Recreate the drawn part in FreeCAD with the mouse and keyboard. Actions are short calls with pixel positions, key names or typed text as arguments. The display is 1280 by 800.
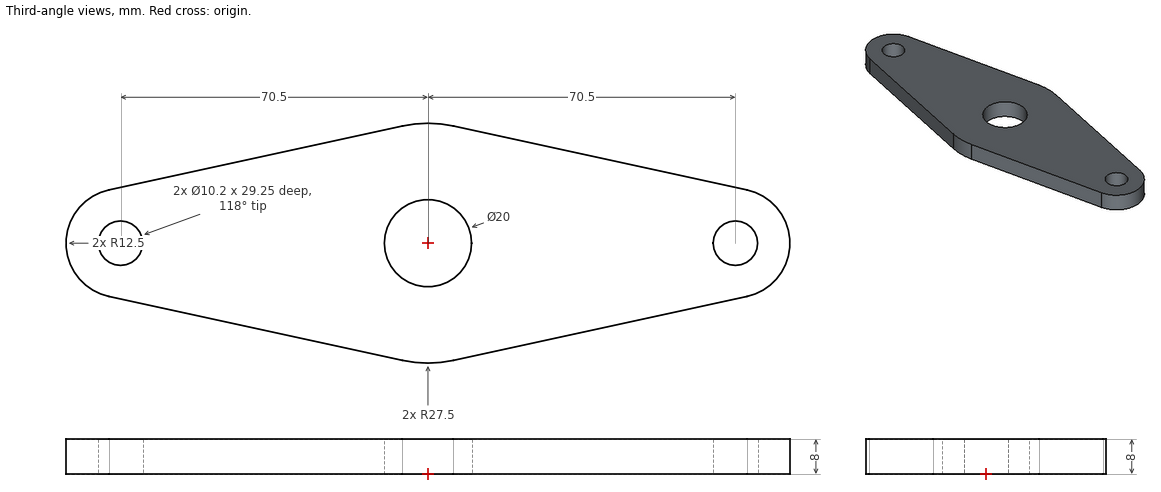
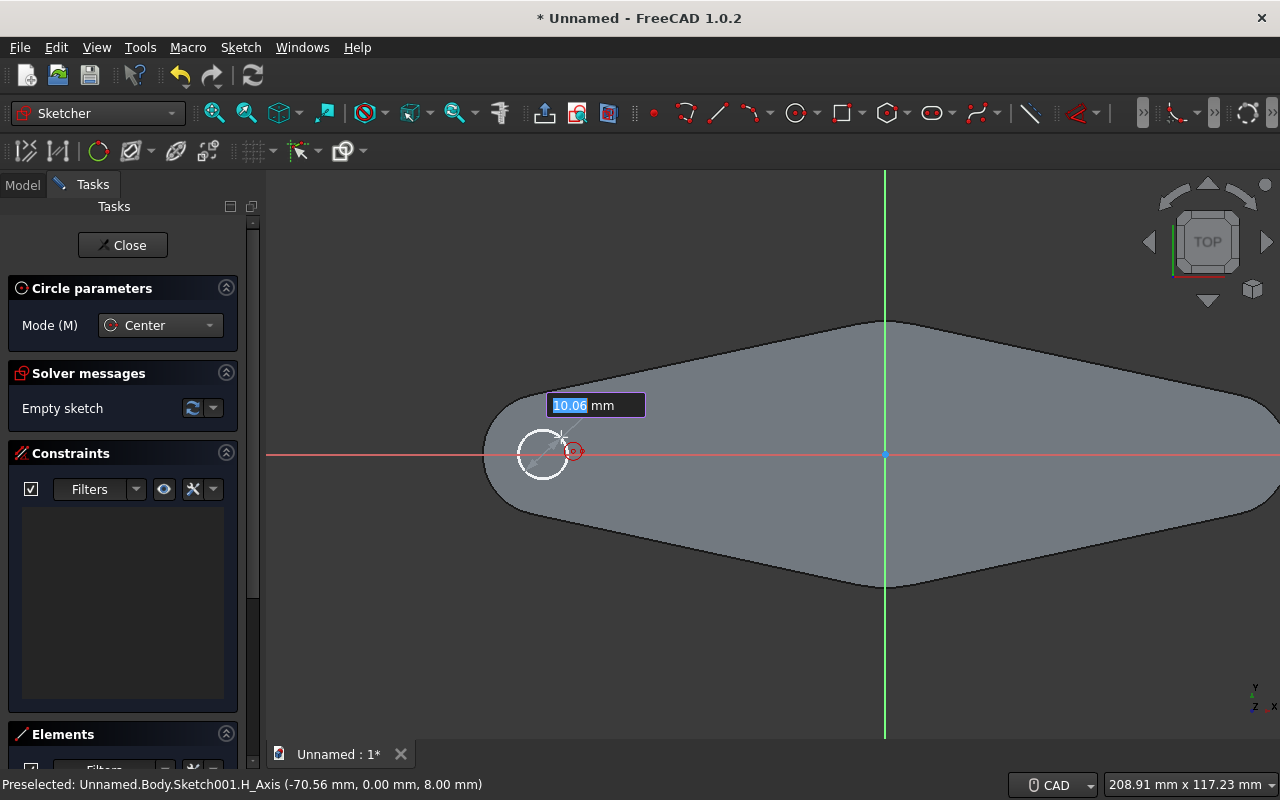
text(10.2)
key(Return)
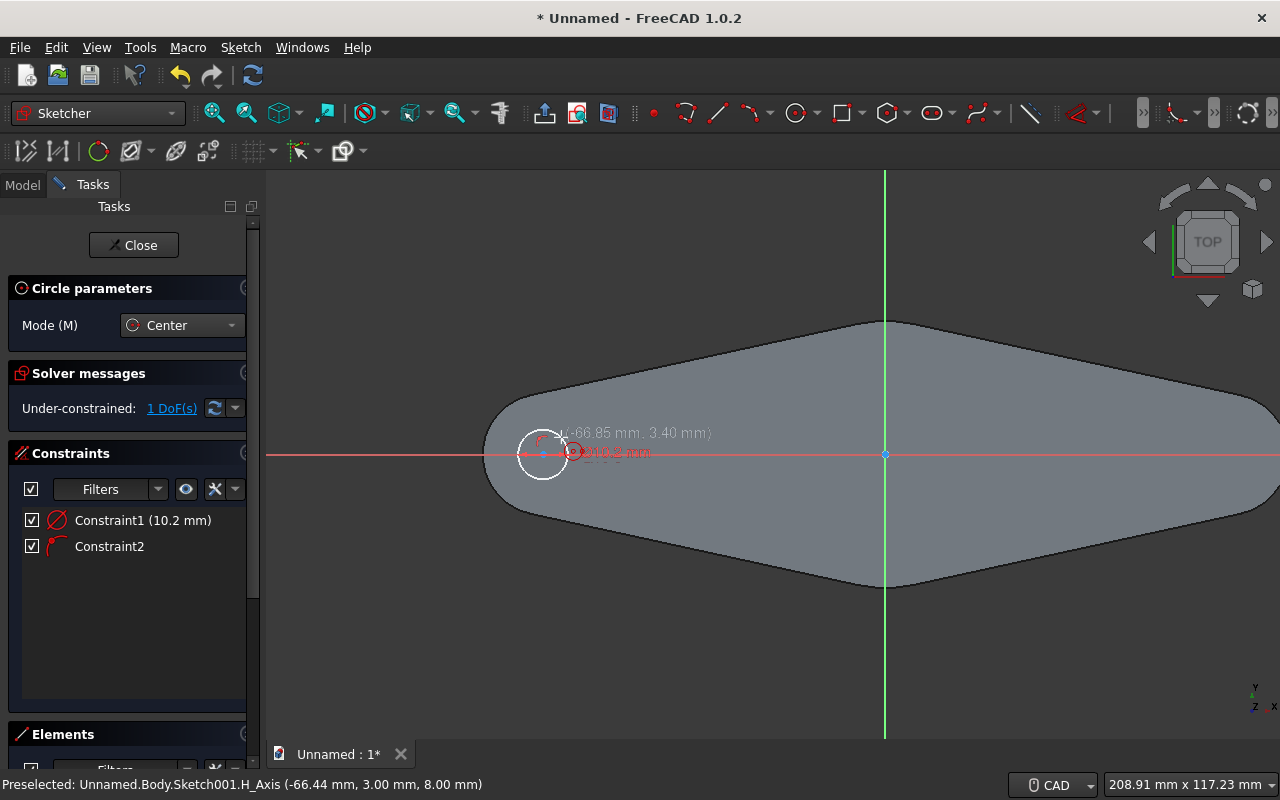
scroll(294, 455, down, 1)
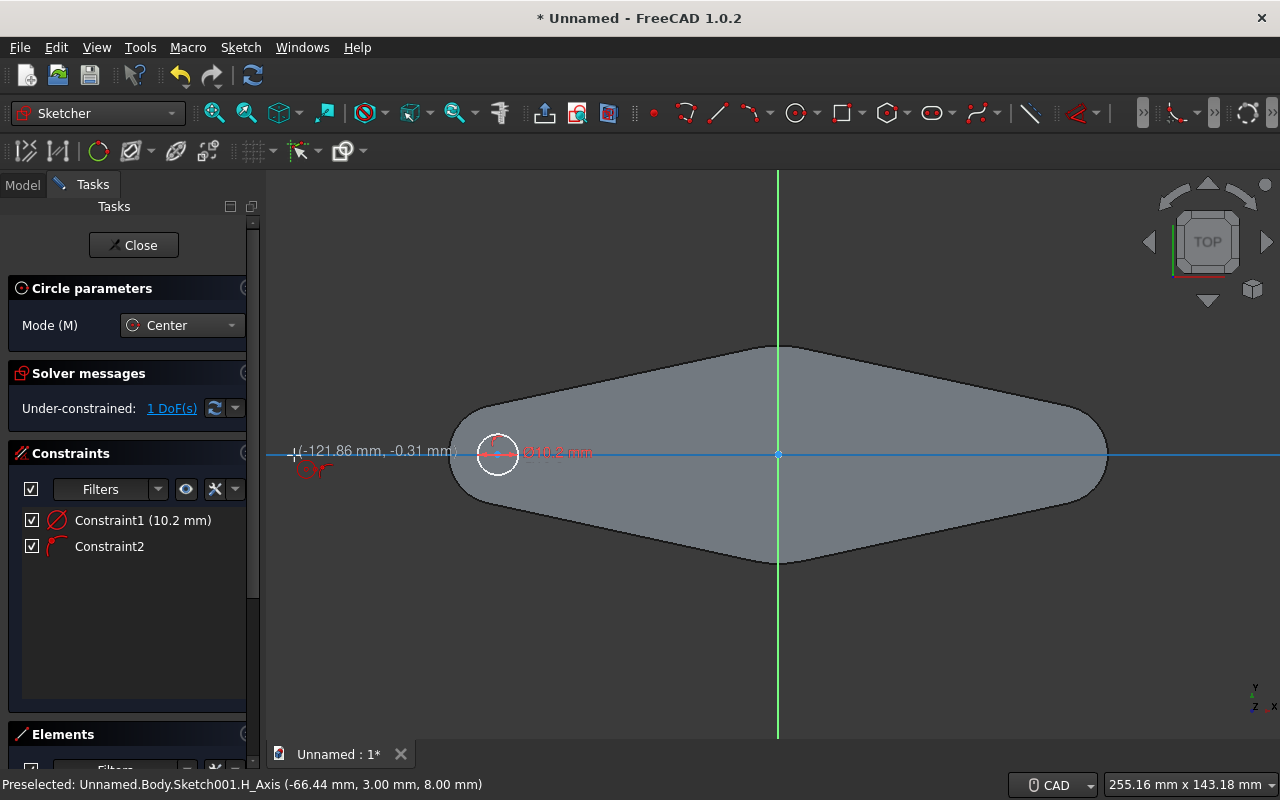
click(1058, 455)
move(1073, 440)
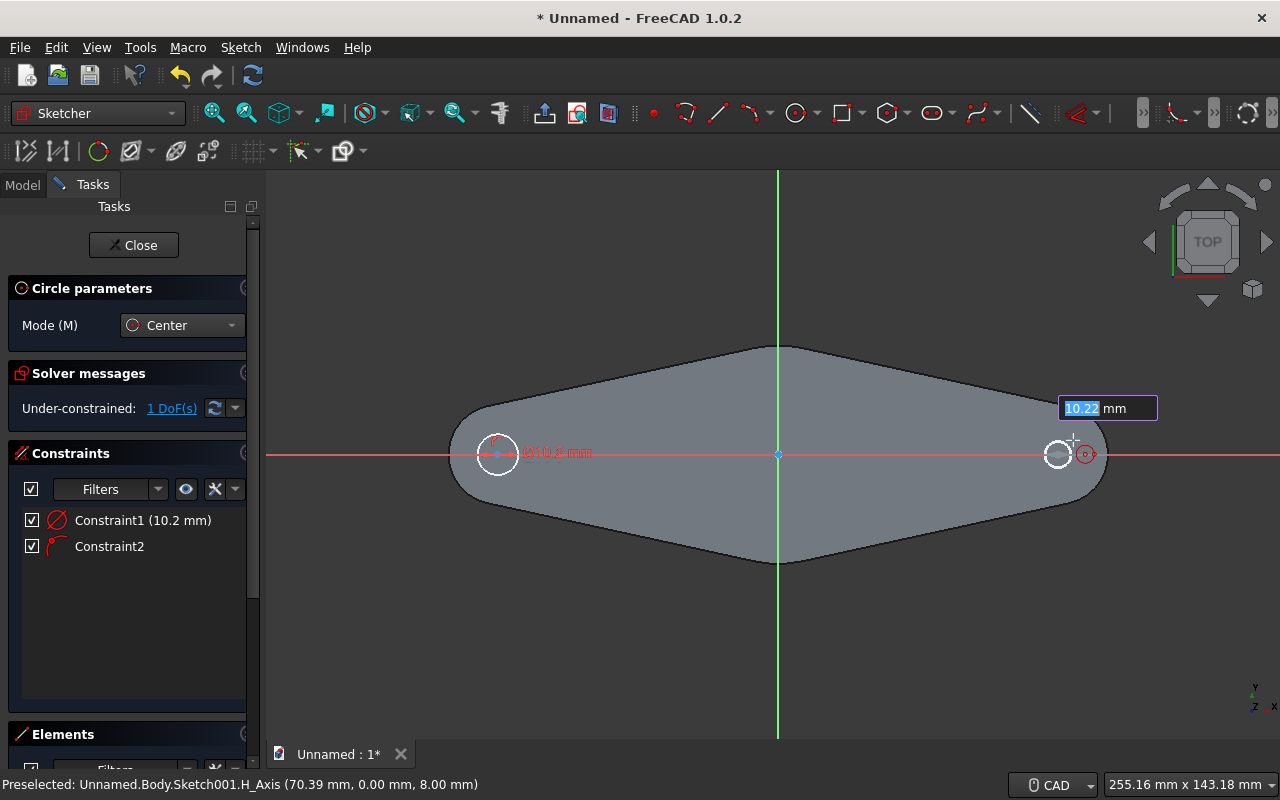
text(10.2)
key(Return)
key(Escape)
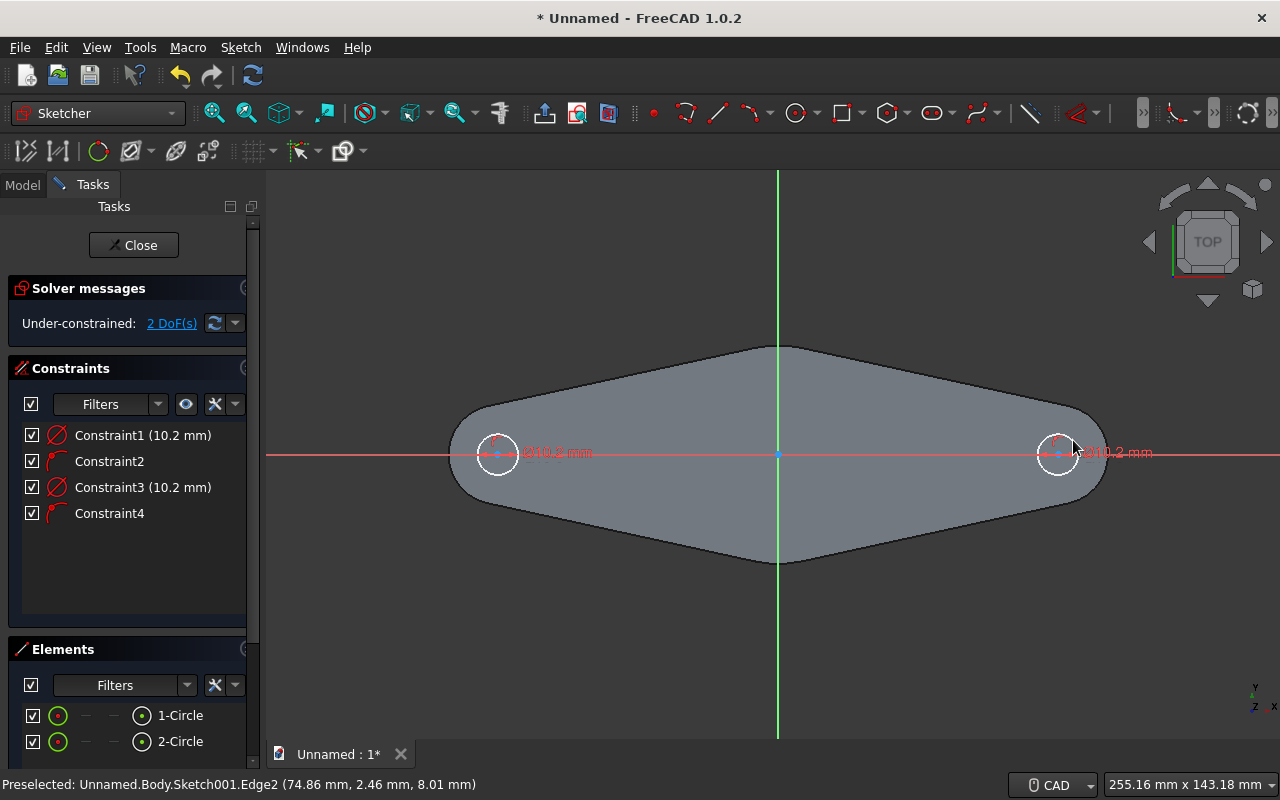
click(498, 455)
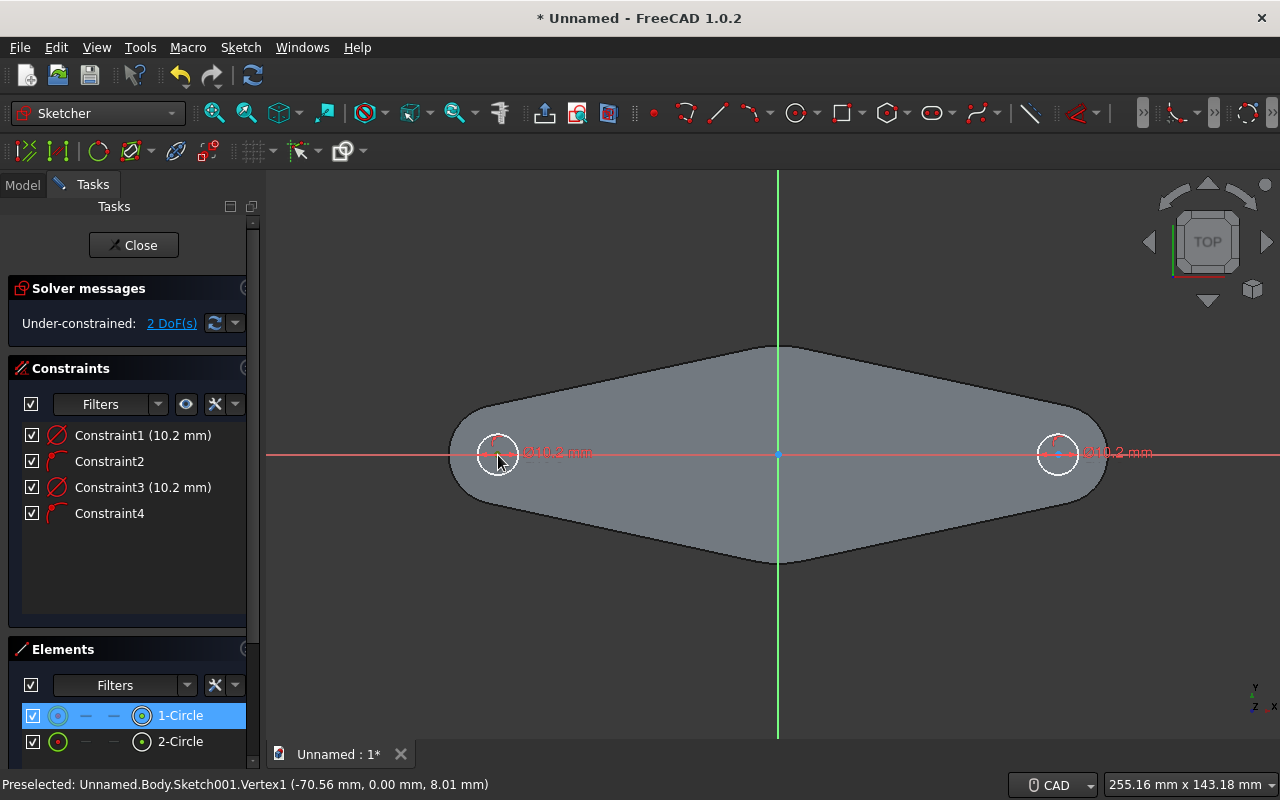
click(1098, 114)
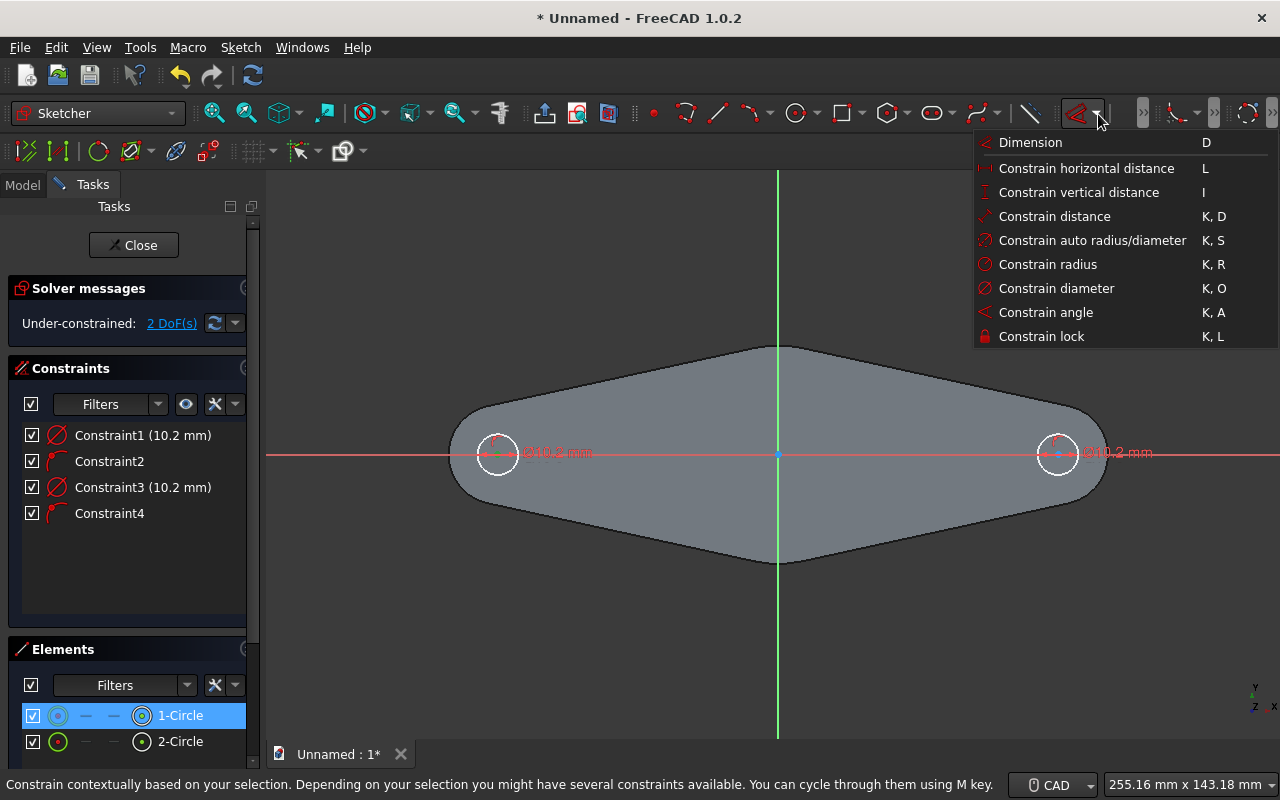
click(1126, 168)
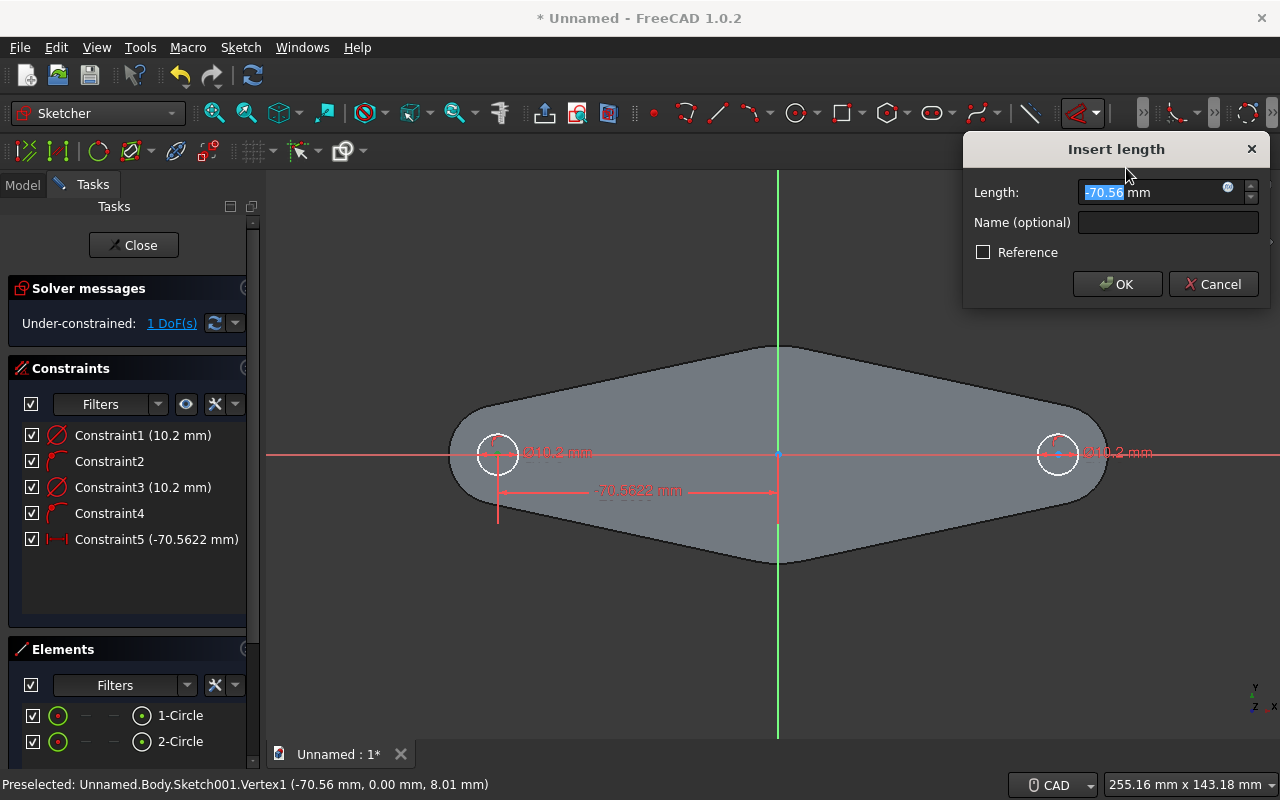
text(-70.5)
key(Return)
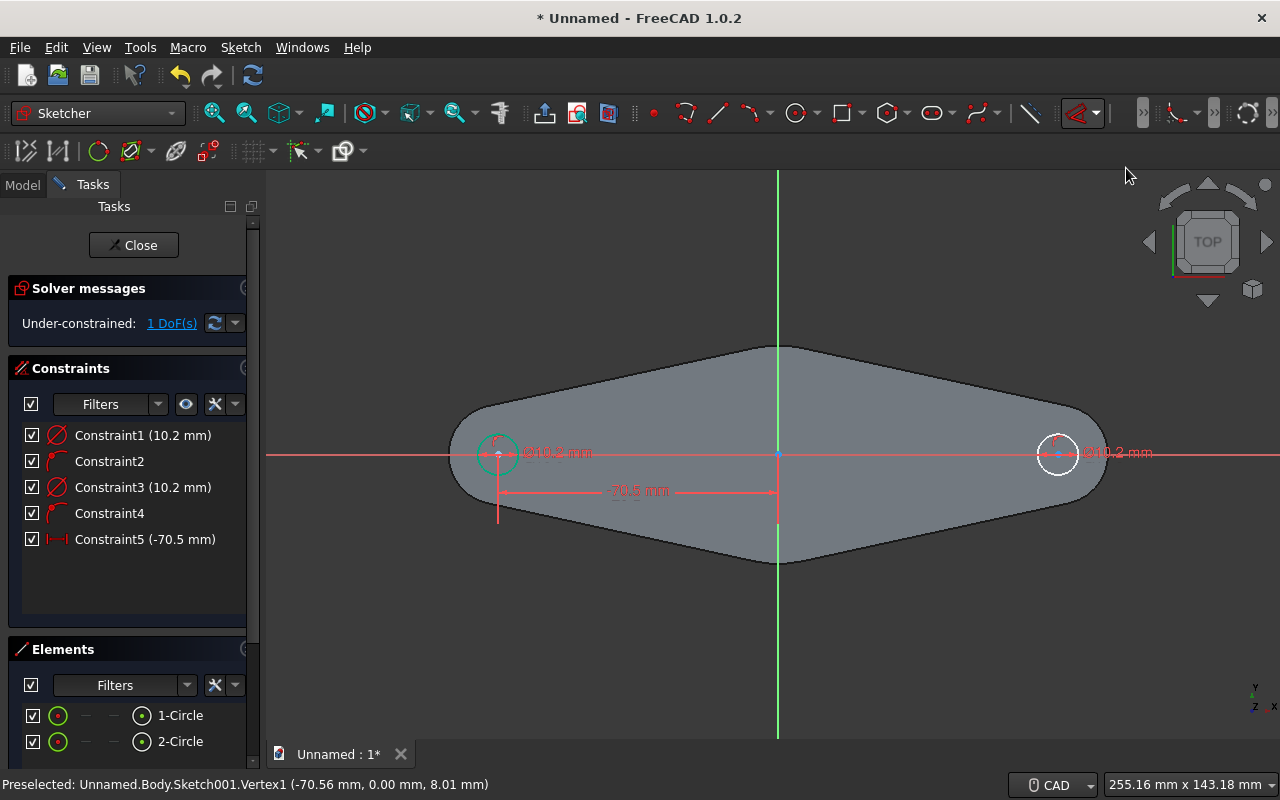
click(1058, 455)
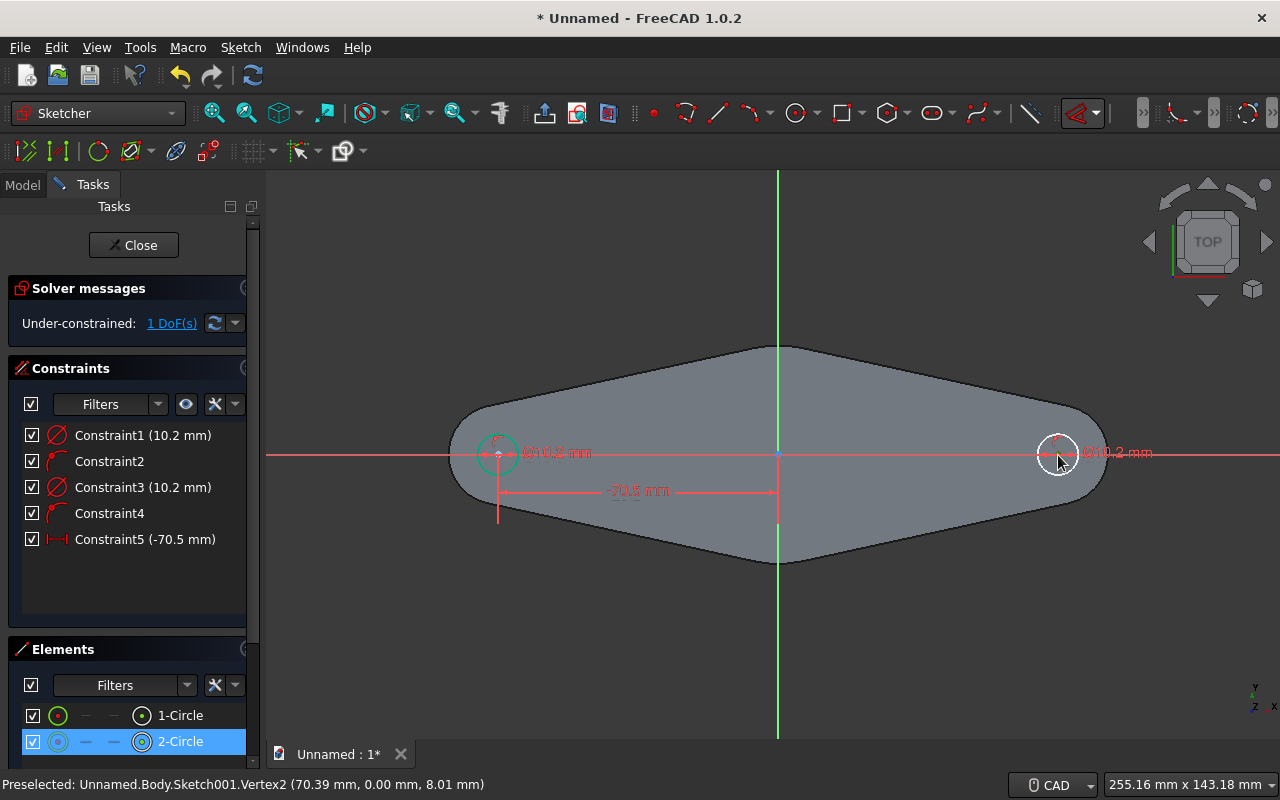
key(l)